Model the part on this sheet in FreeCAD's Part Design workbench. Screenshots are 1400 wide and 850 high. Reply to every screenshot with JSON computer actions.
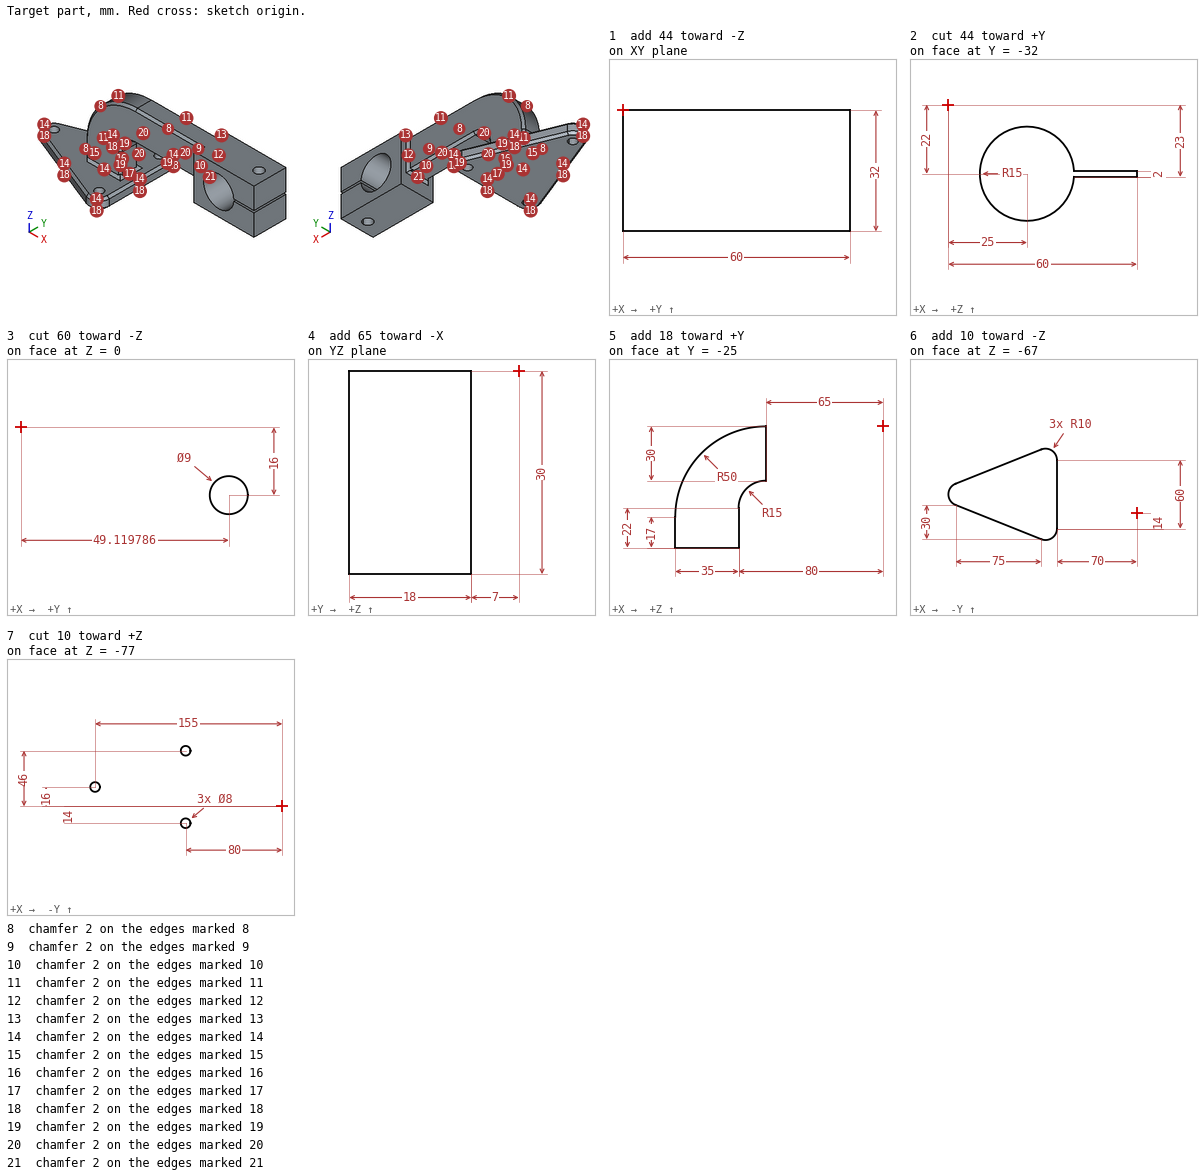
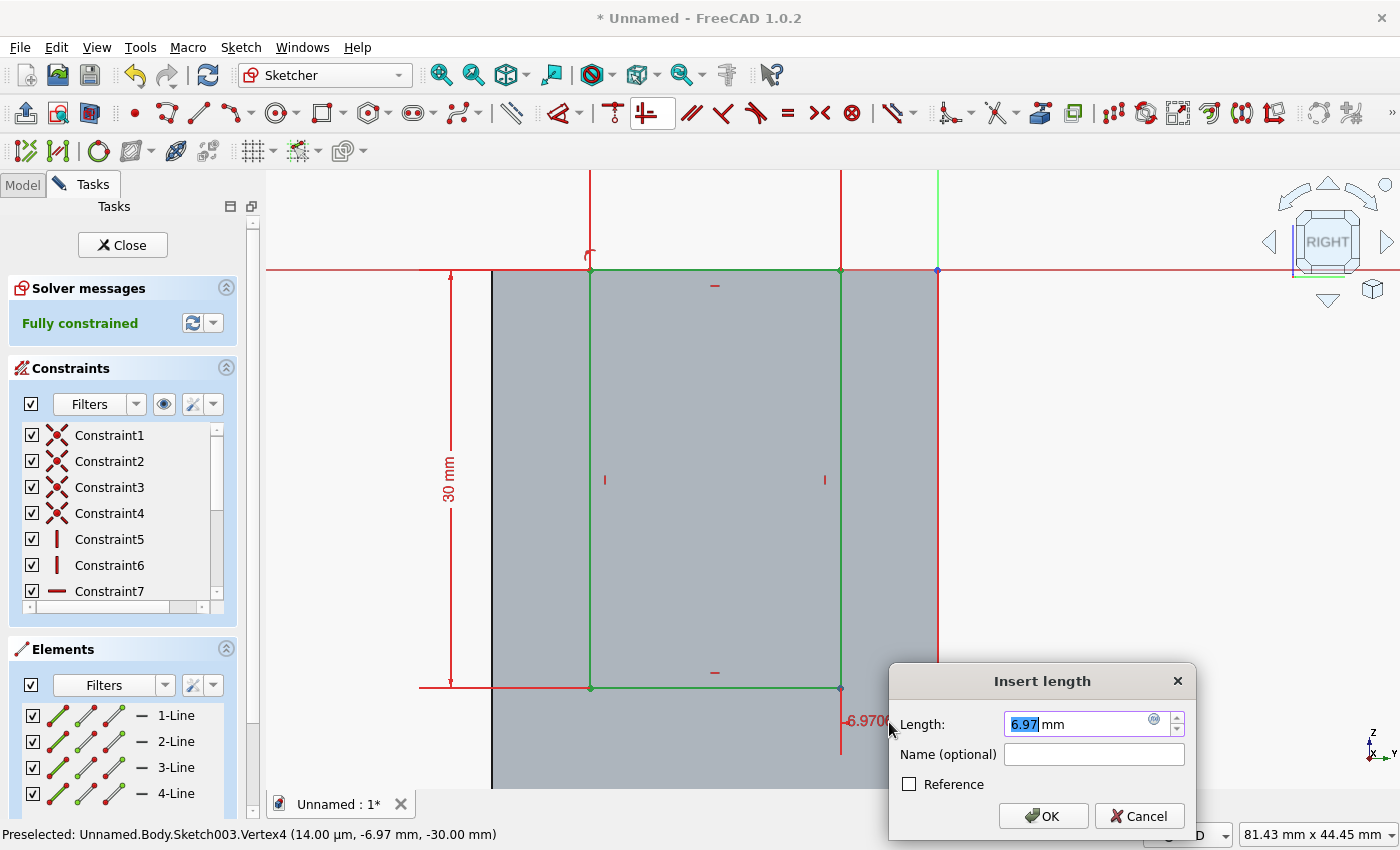
{"action": "type", "text": "7"}
{"action": "key", "text": "Return"}
{"action": "key", "text": "Escape"}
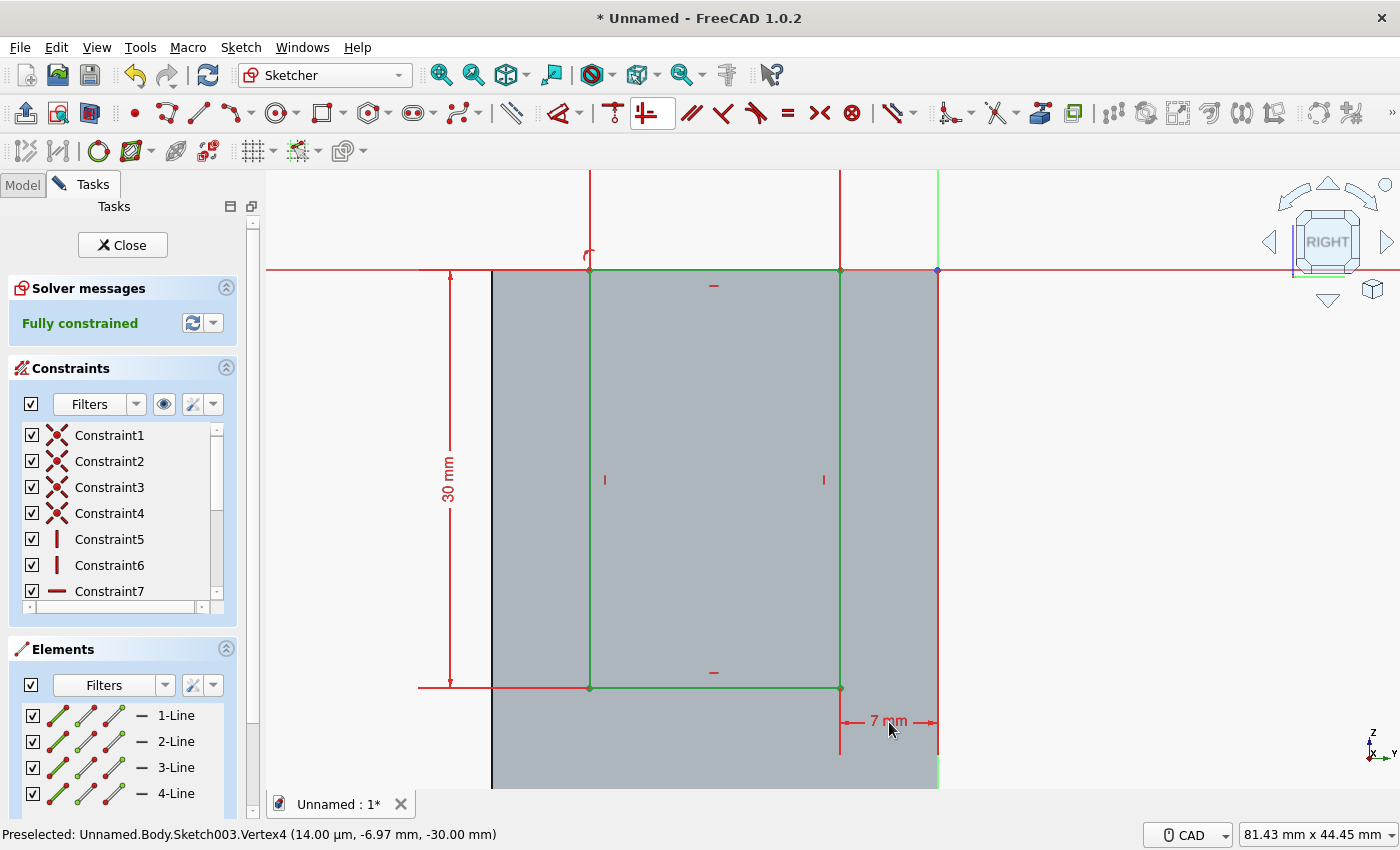
{"action": "left_click", "coordinate": [123, 245]}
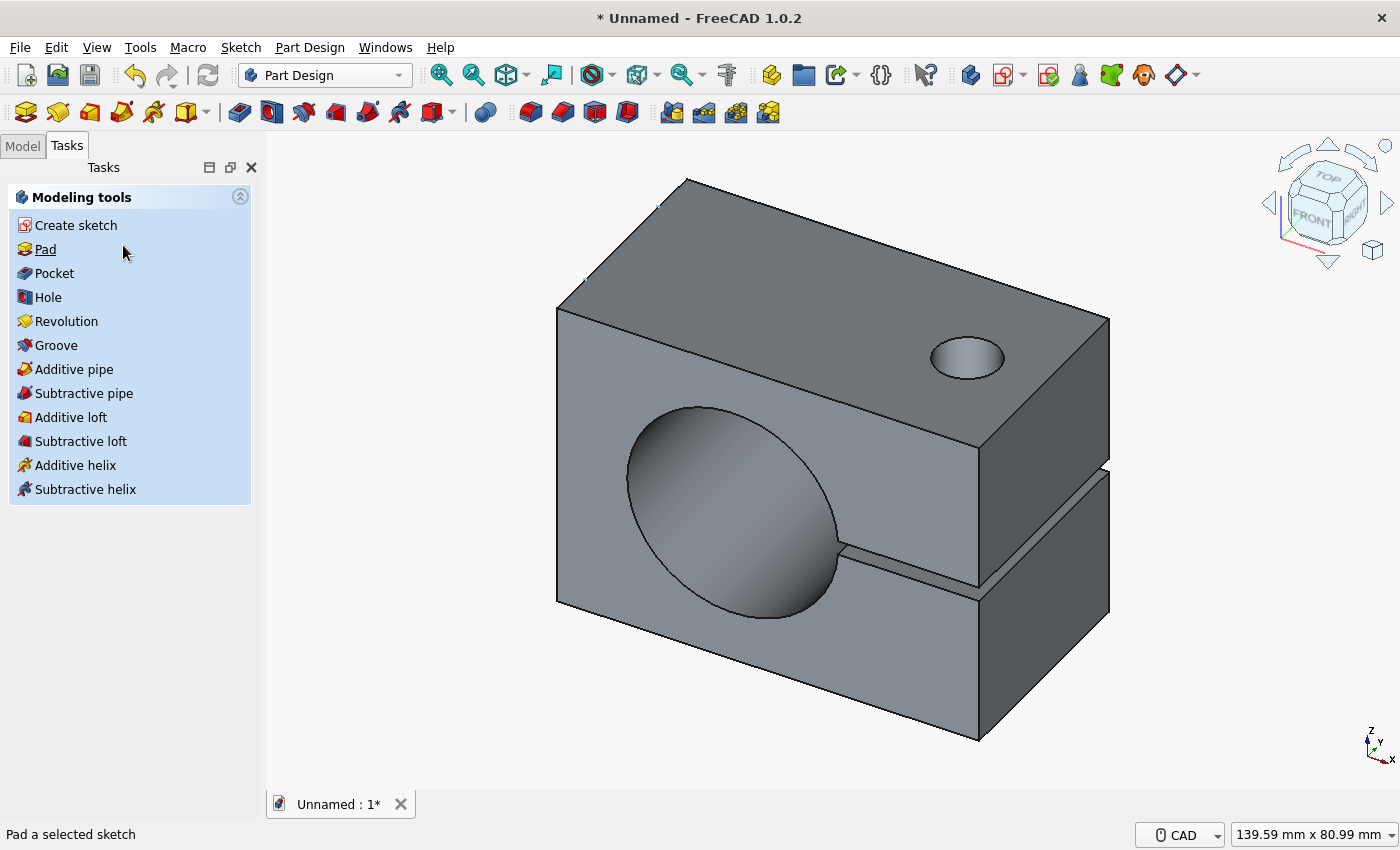
{"action": "left_click", "coordinate": [26, 112]}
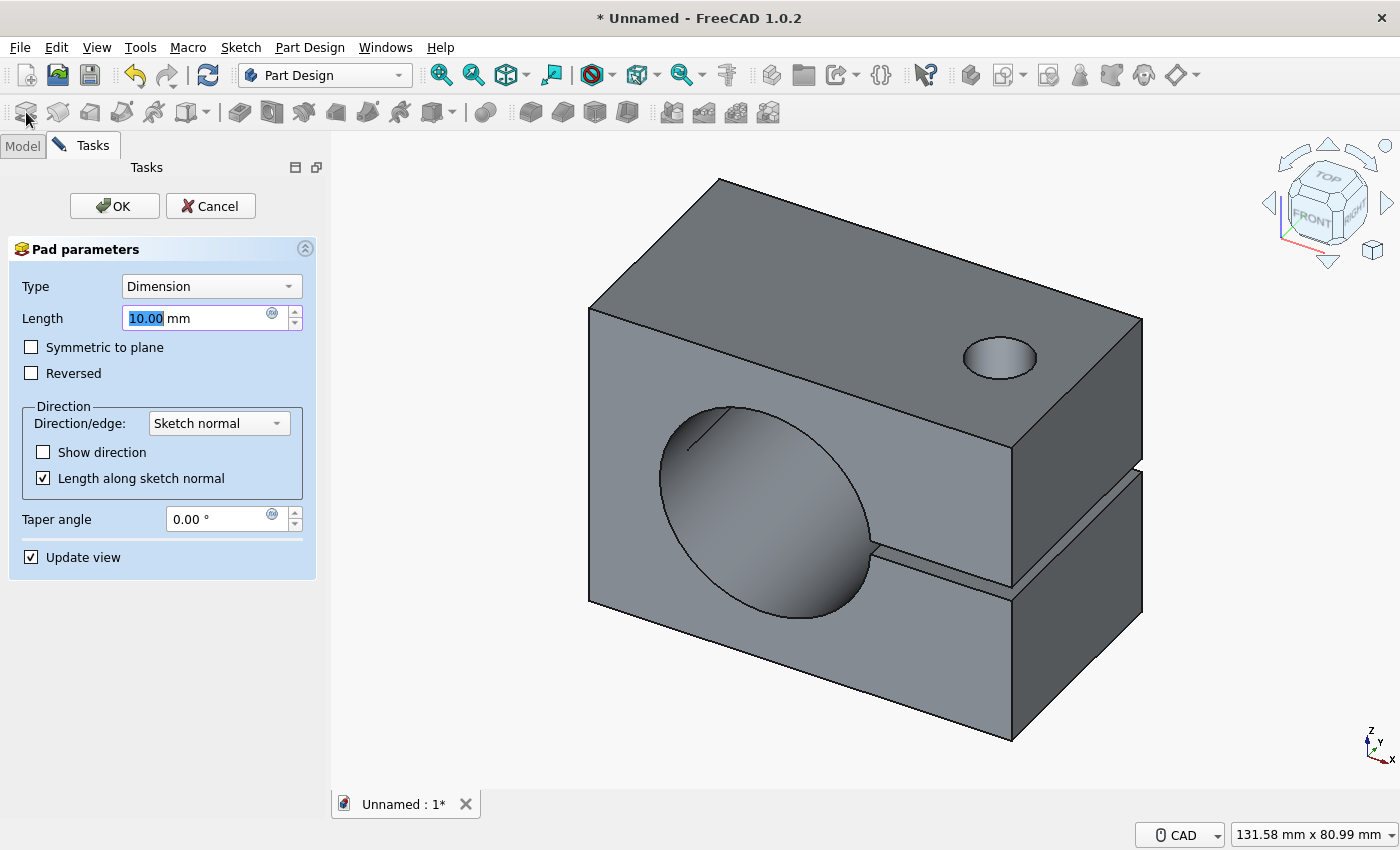
{"action": "type", "text": "65"}
{"action": "key", "text": "Tab"}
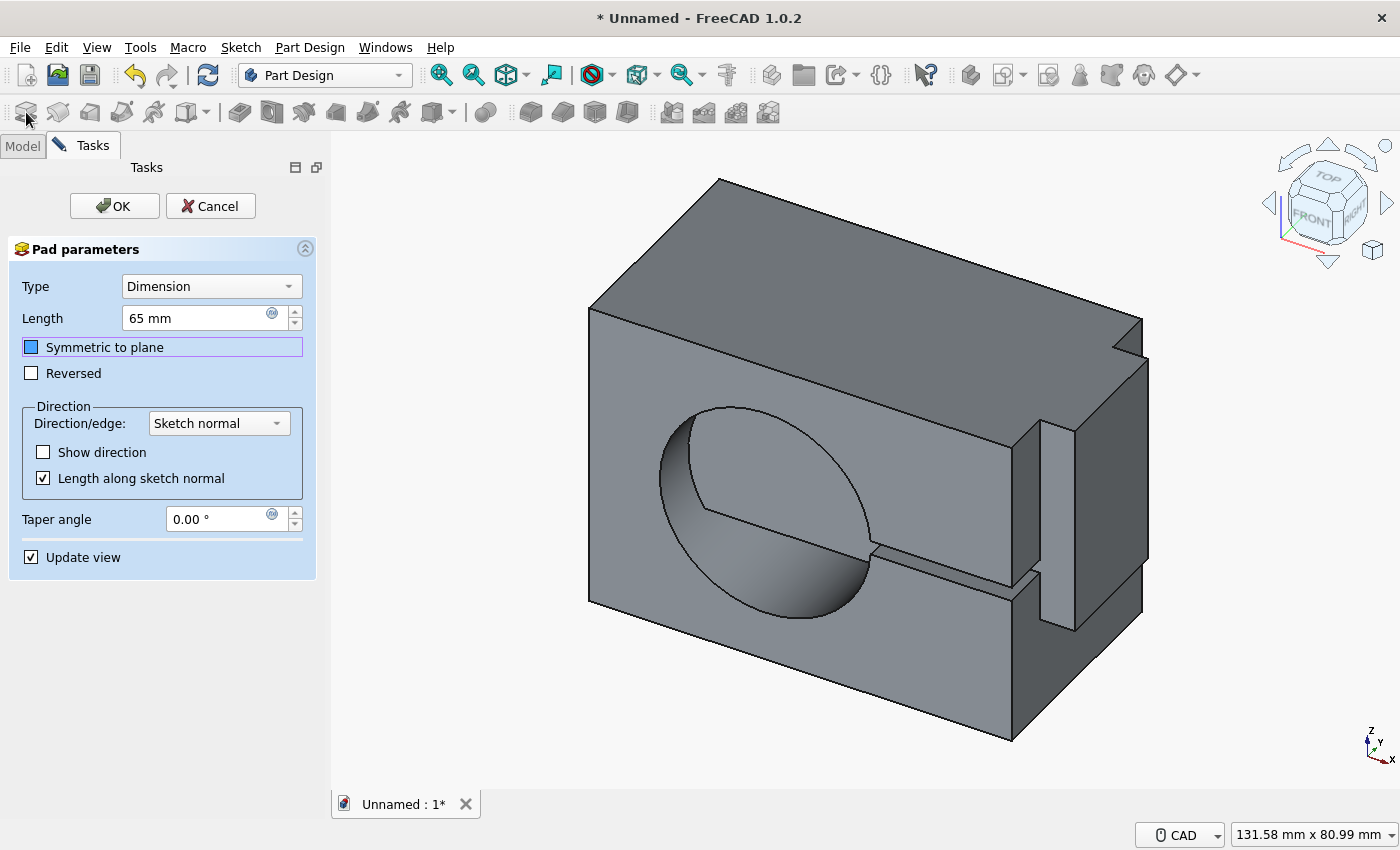
{"action": "left_click", "coordinate": [30, 373]}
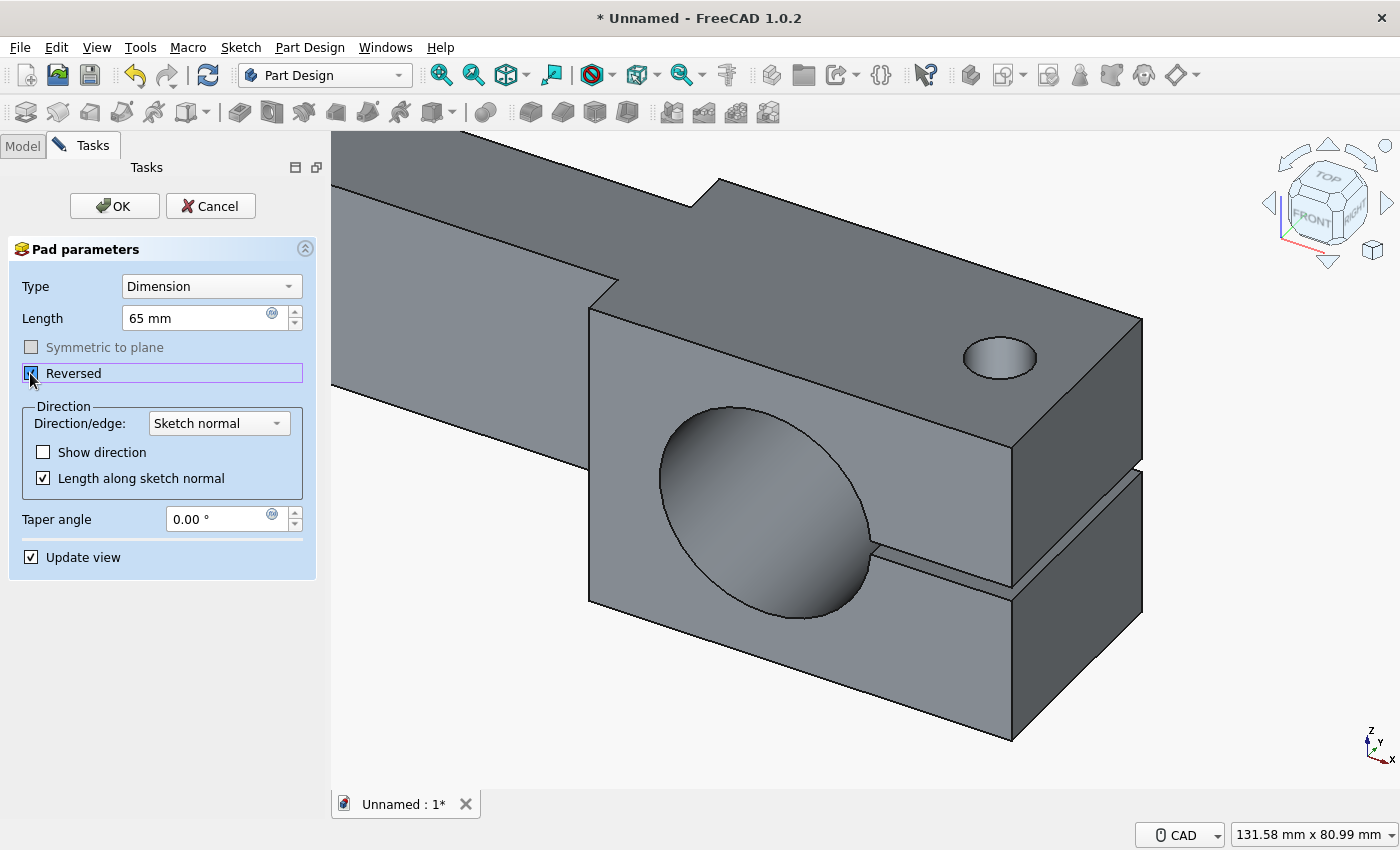
{"action": "left_click", "coordinate": [115, 206]}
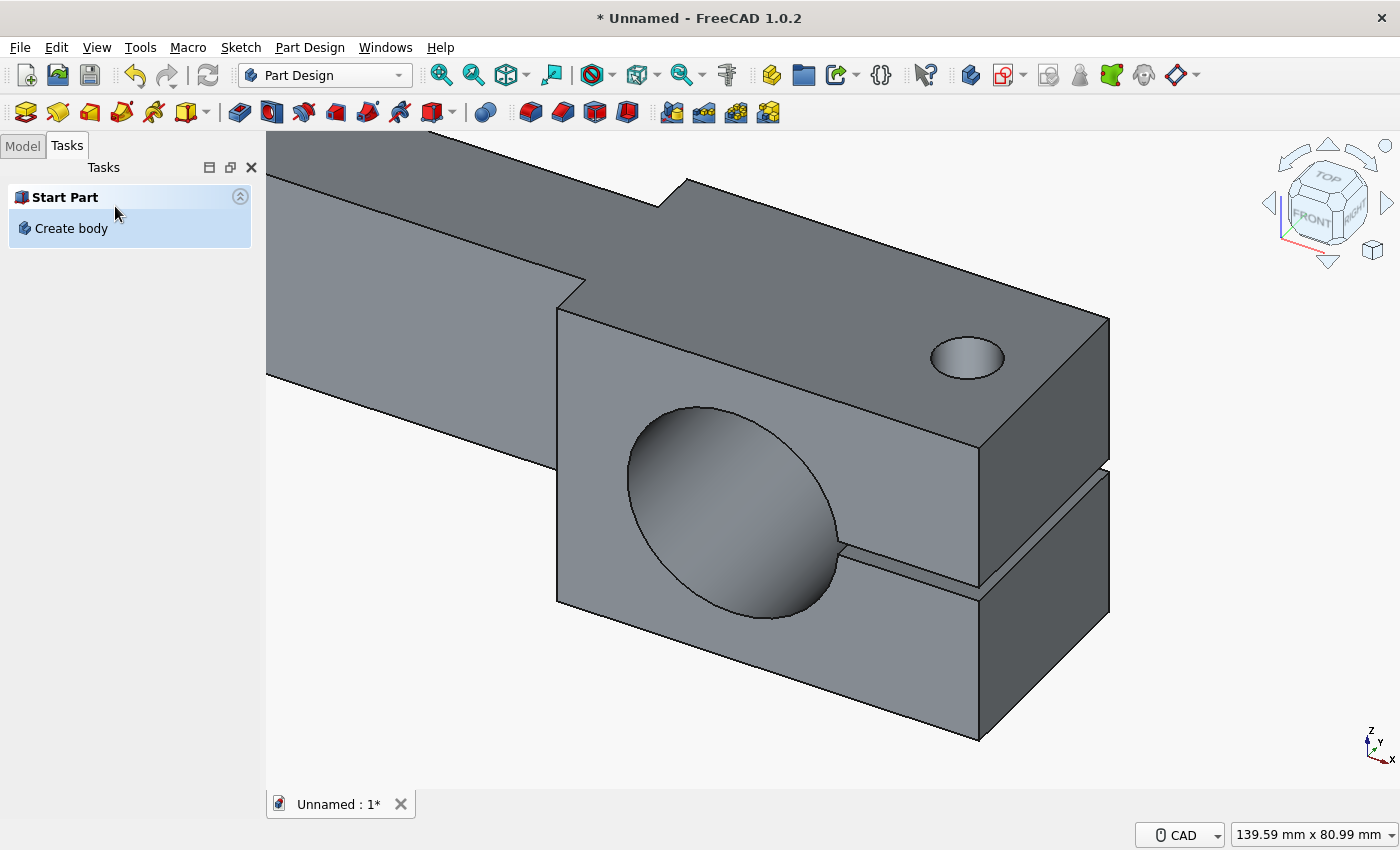
{"action": "left_click", "coordinate": [442, 76]}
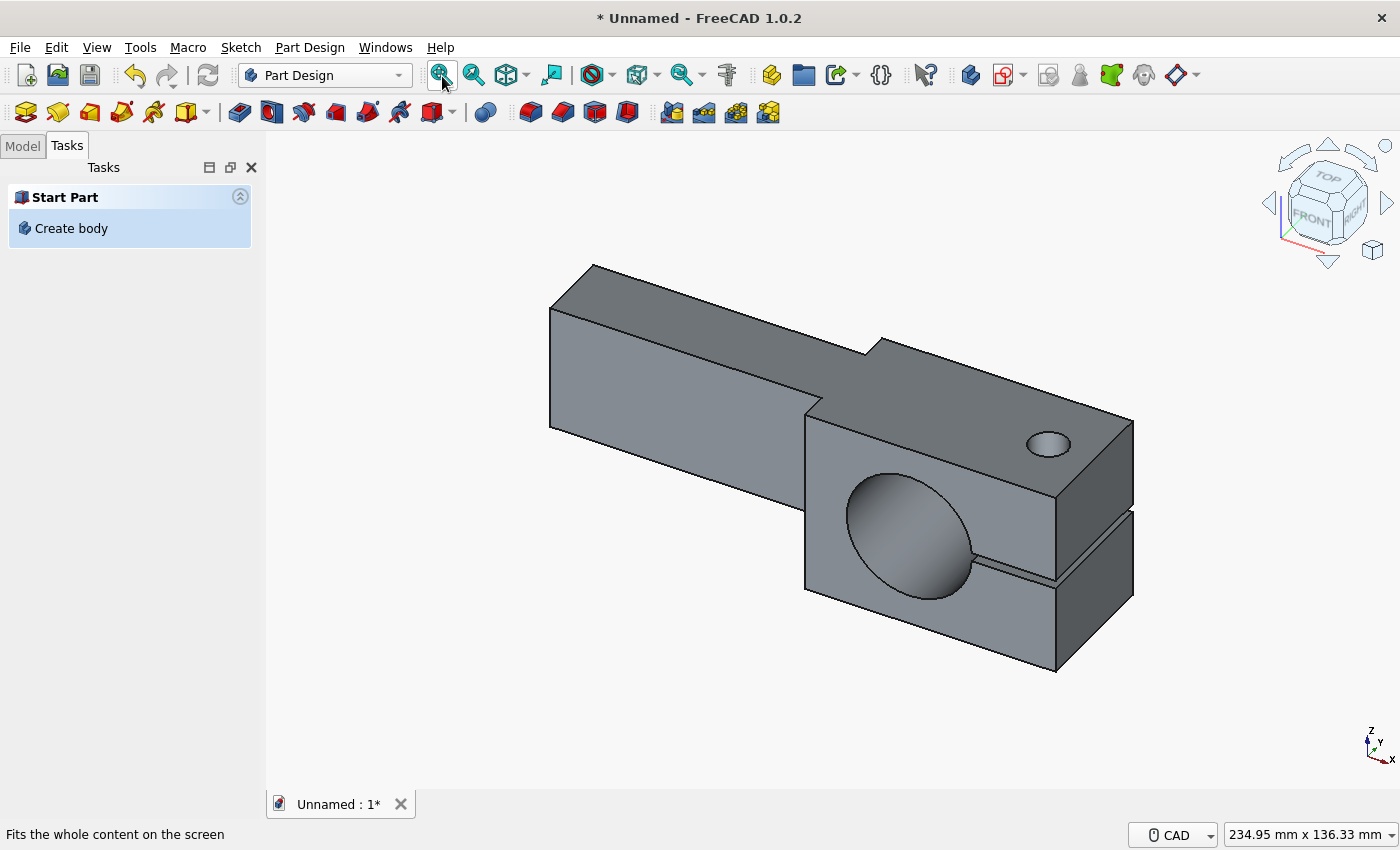
{"action": "left_click", "coordinate": [725, 424]}